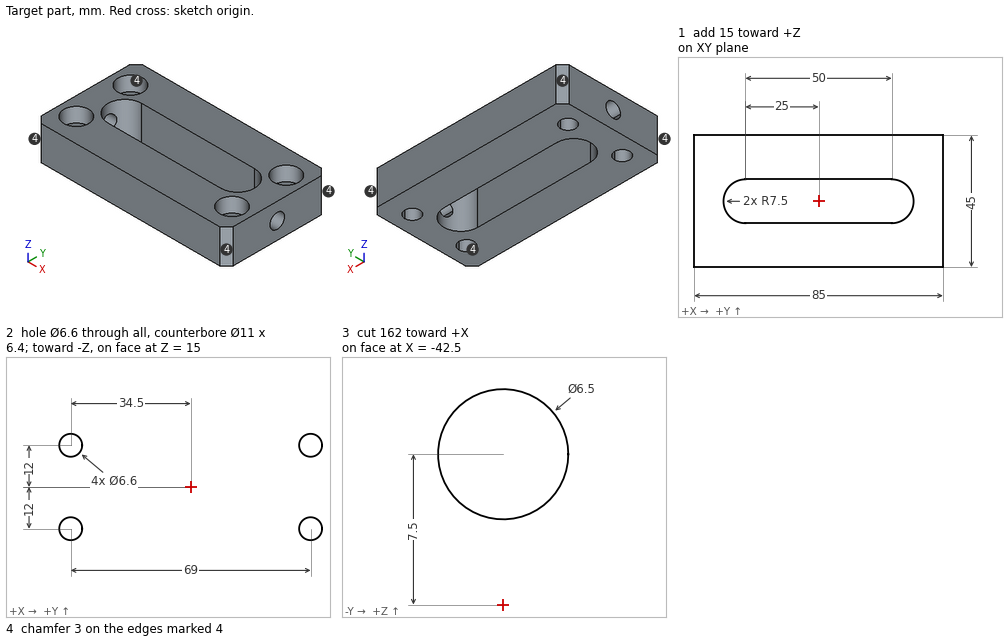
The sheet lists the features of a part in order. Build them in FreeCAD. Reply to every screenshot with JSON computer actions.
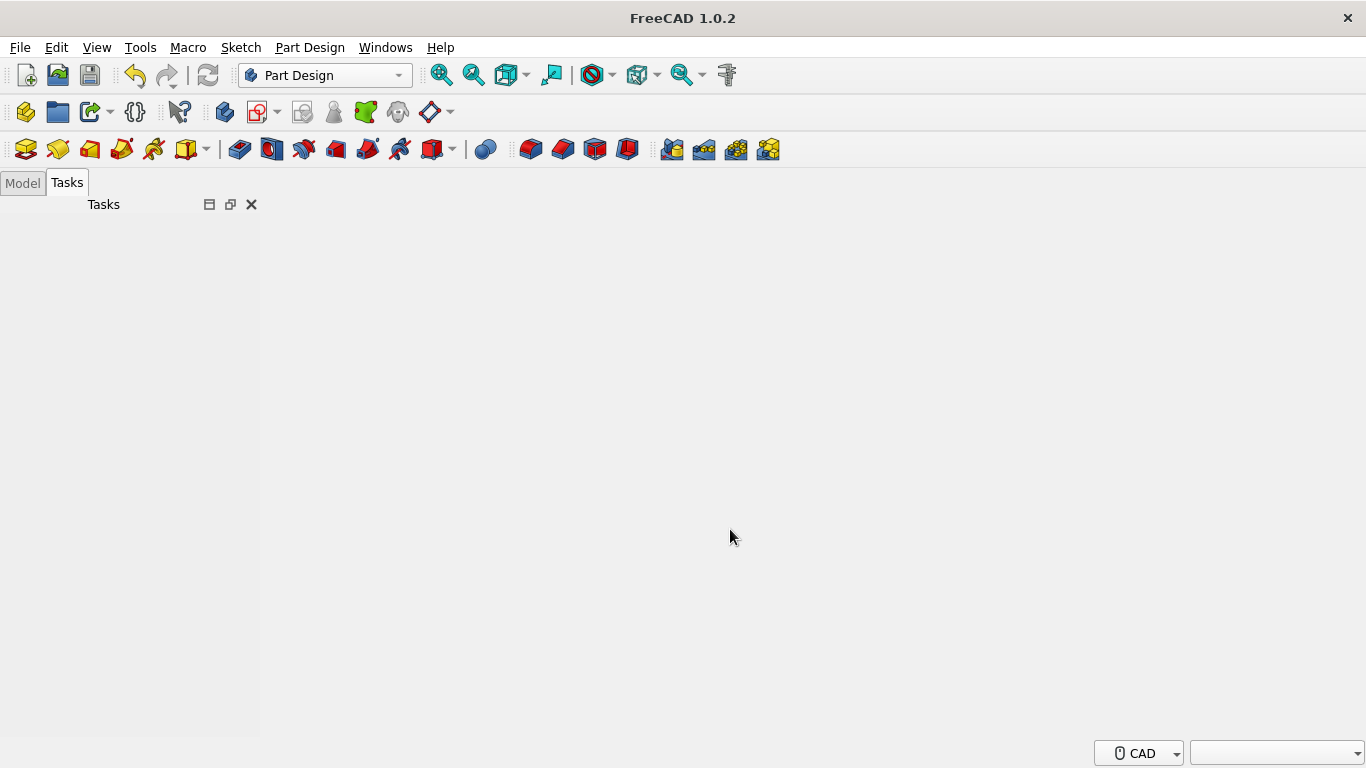
{"action": "key", "text": "ctrl+n"}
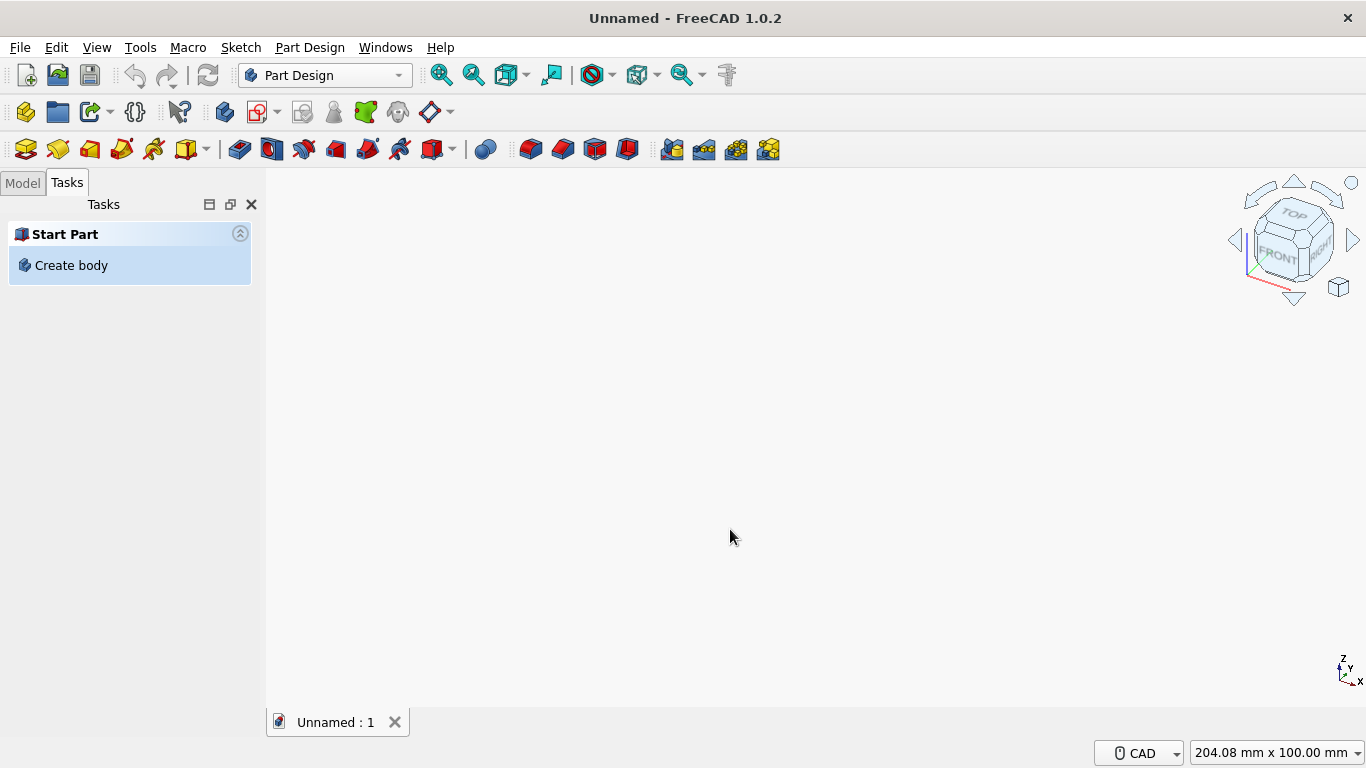
{"action": "left_click", "coordinate": [258, 112]}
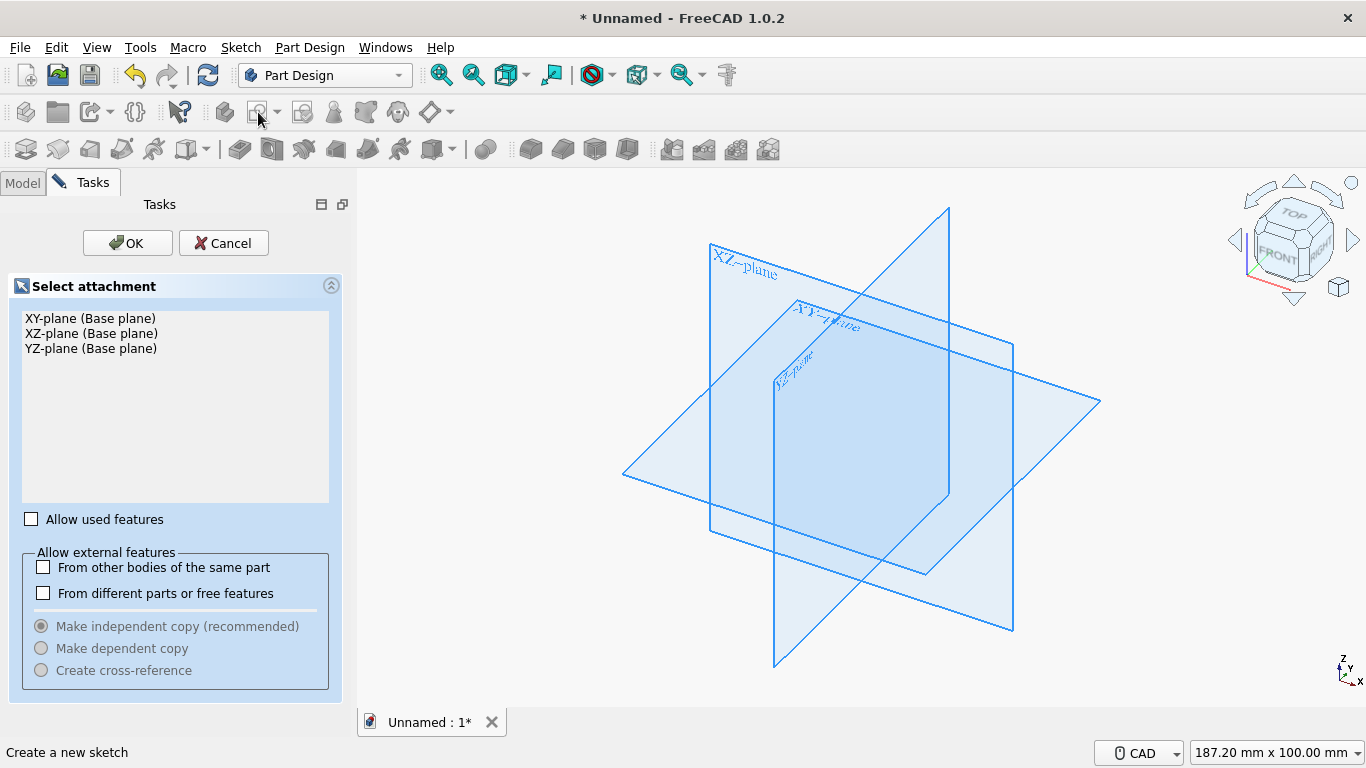
{"action": "left_click", "coordinate": [82, 318]}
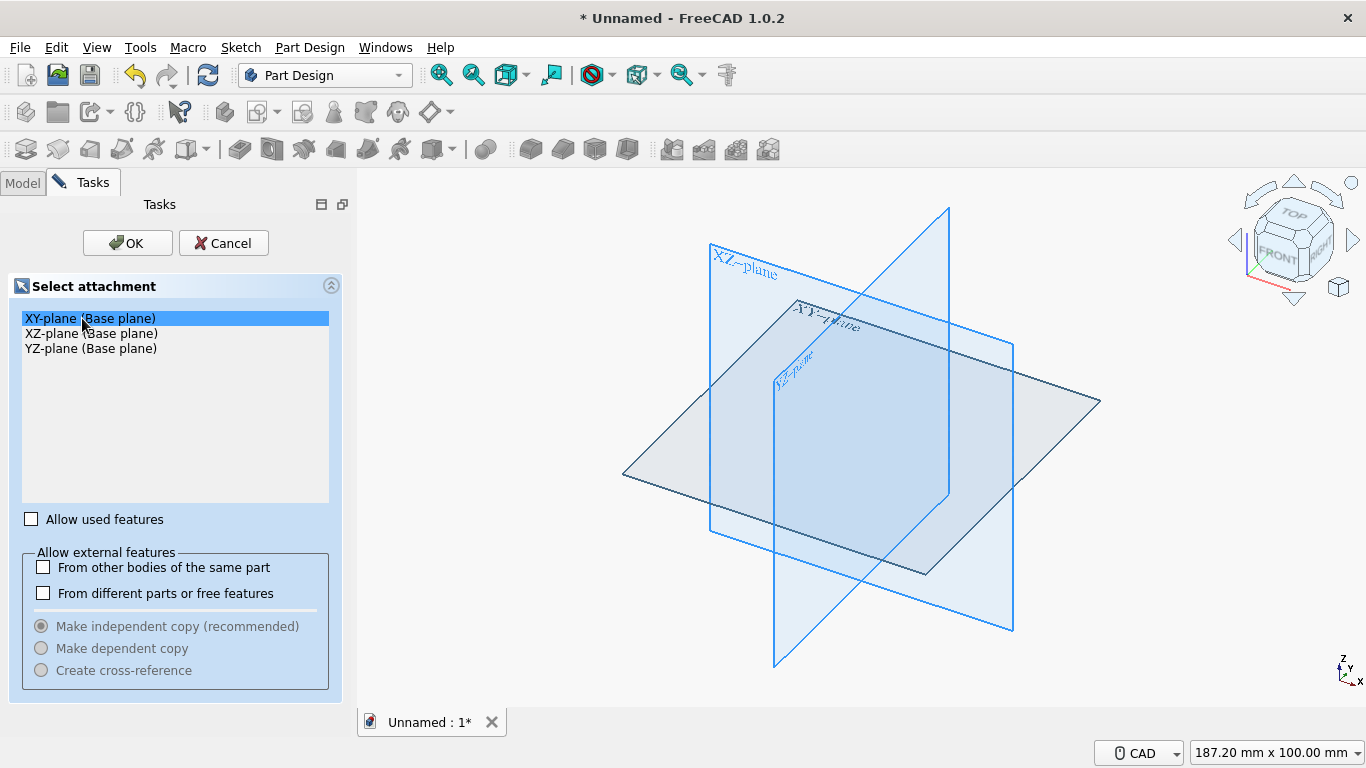
{"action": "left_click", "coordinate": [128, 243]}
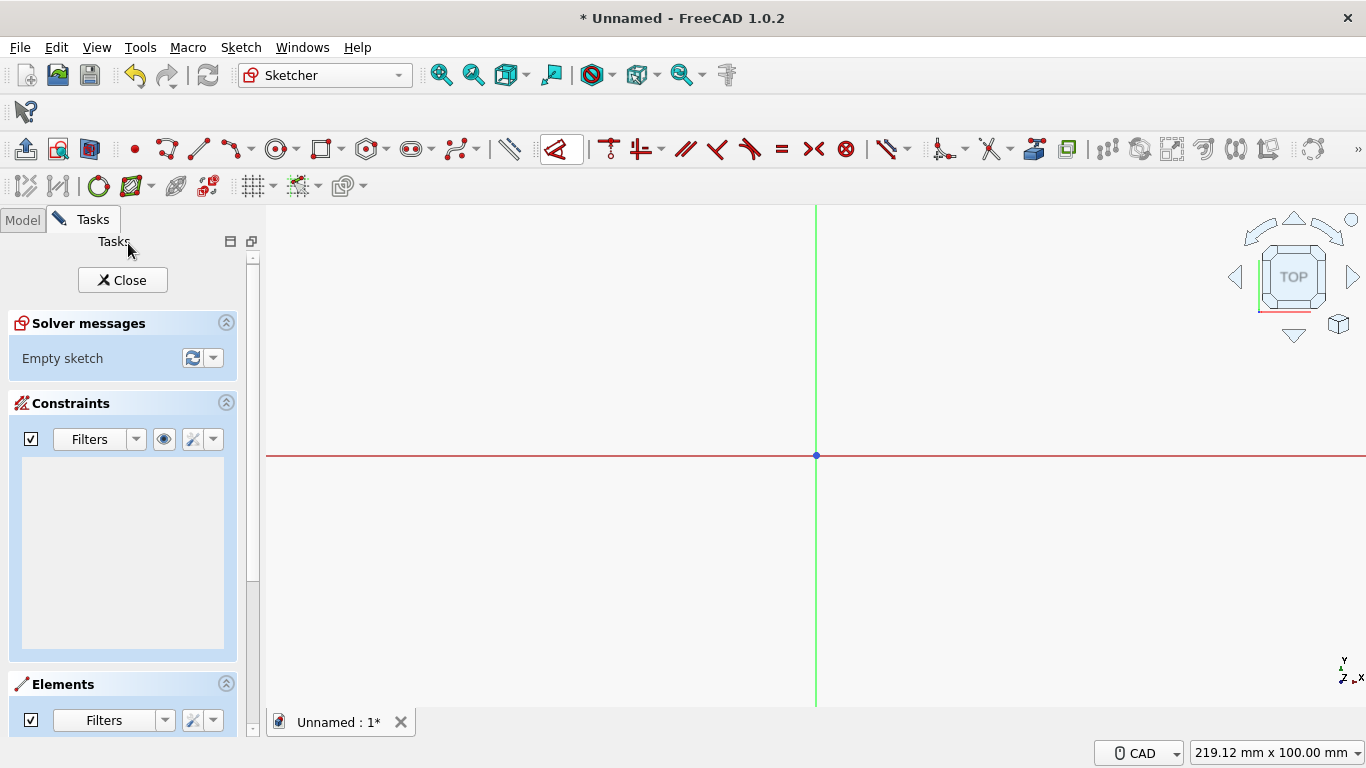
{"action": "scroll", "coordinate": [955, 456], "scroll_direction": "up", "scroll_amount": 2}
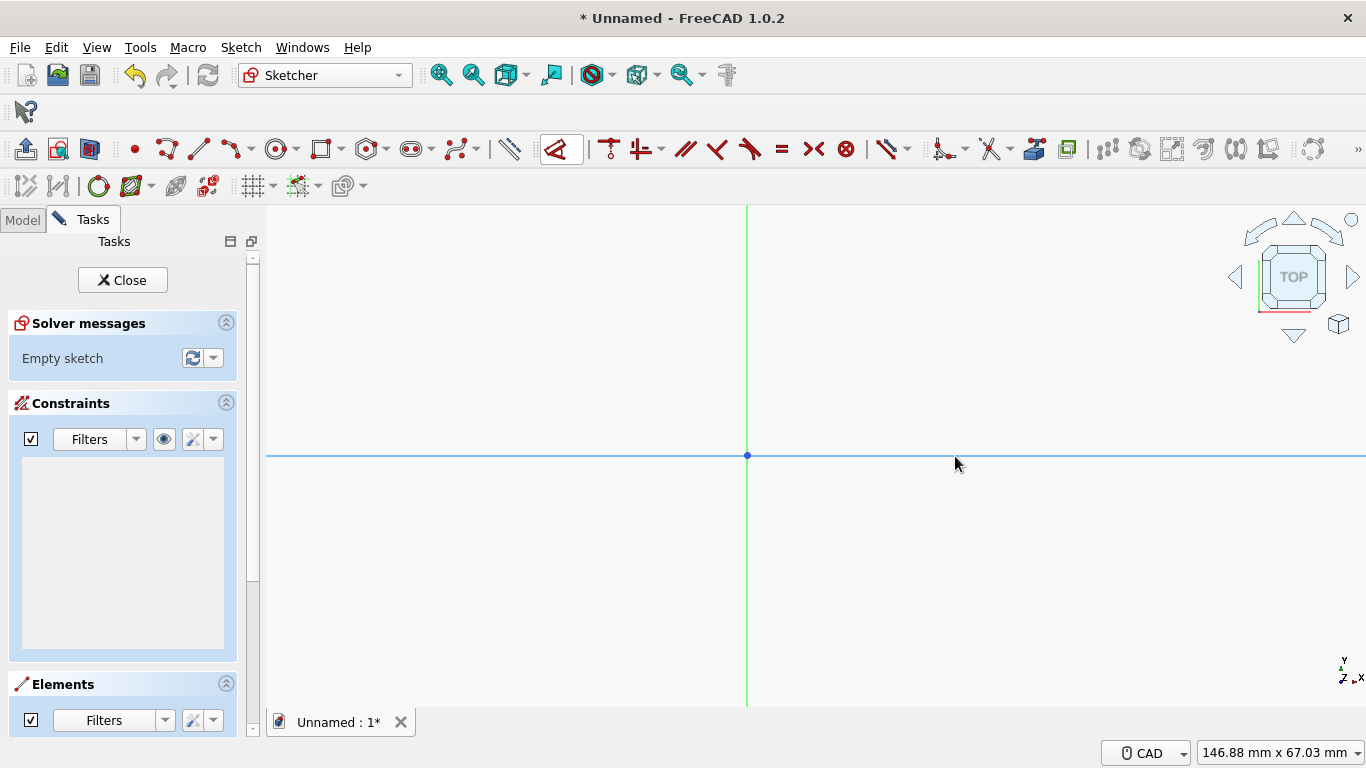
{"action": "key", "text": "g v"}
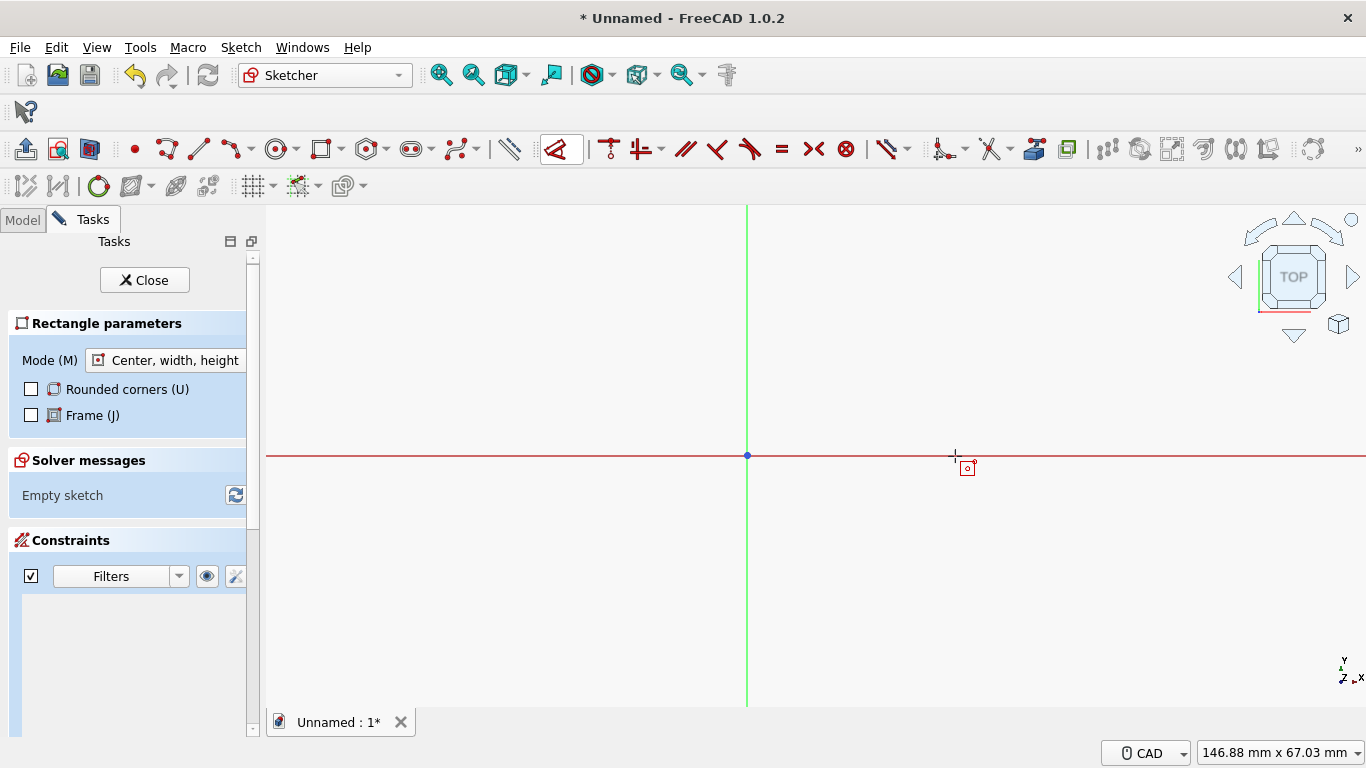
{"action": "left_click", "coordinate": [747, 456]}
{"action": "left_click", "coordinate": [1066, 287]}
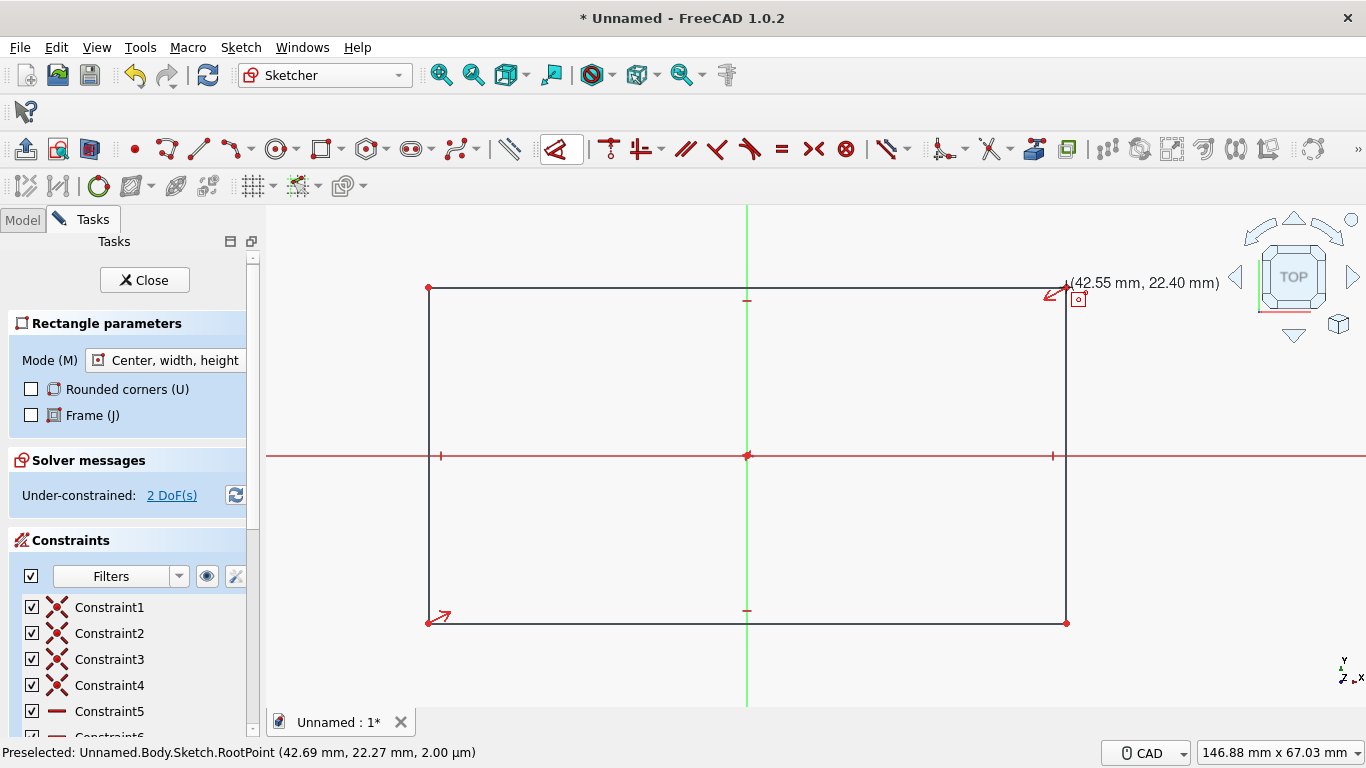
{"action": "left_click", "coordinate": [412, 150]}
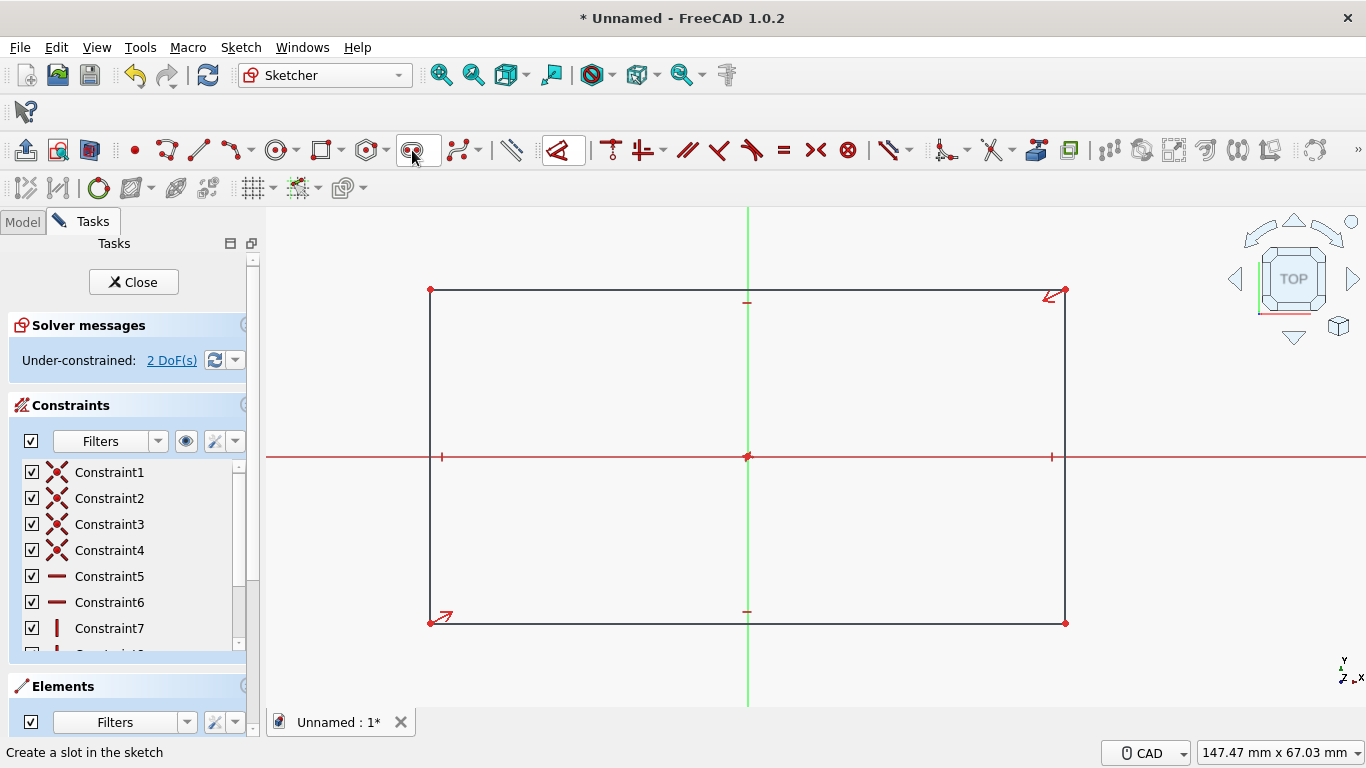
{"action": "left_click", "coordinate": [561, 457]}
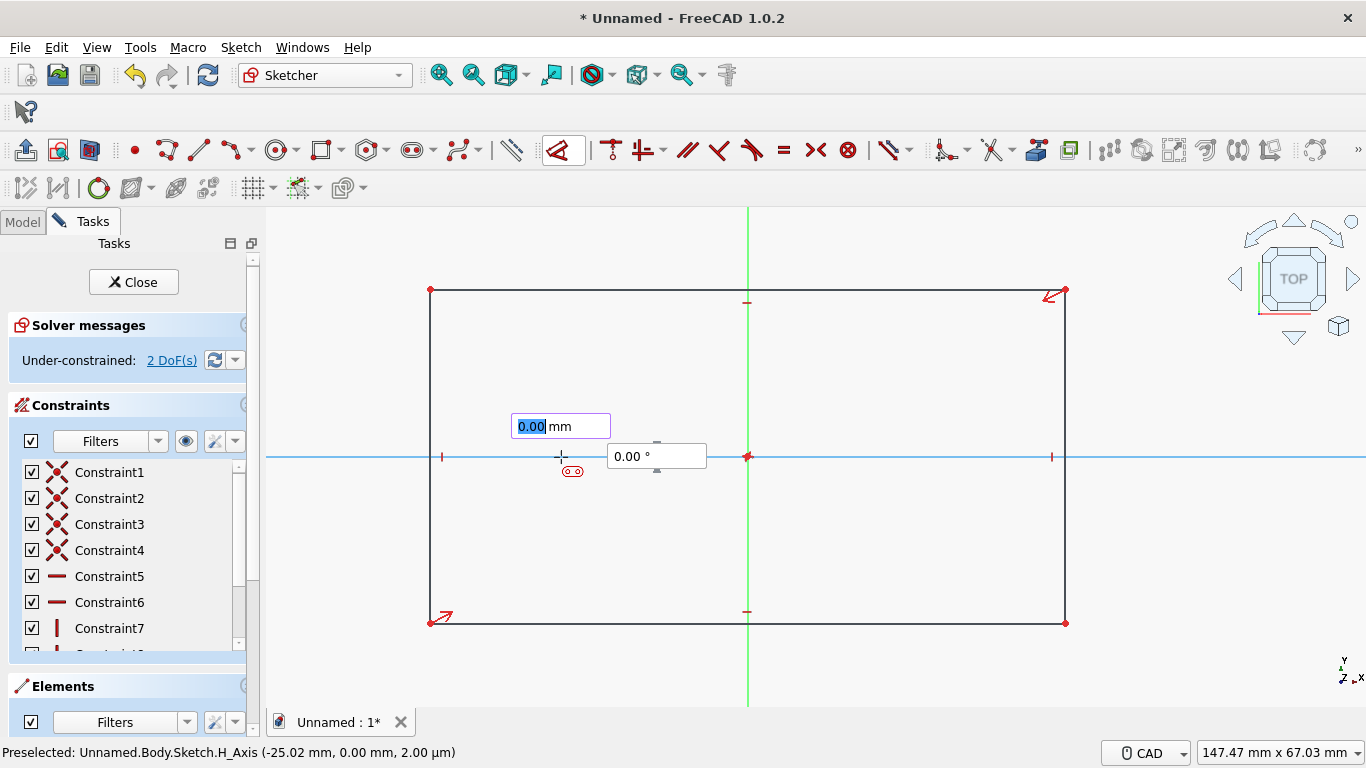
{"action": "left_click", "coordinate": [934, 448]}